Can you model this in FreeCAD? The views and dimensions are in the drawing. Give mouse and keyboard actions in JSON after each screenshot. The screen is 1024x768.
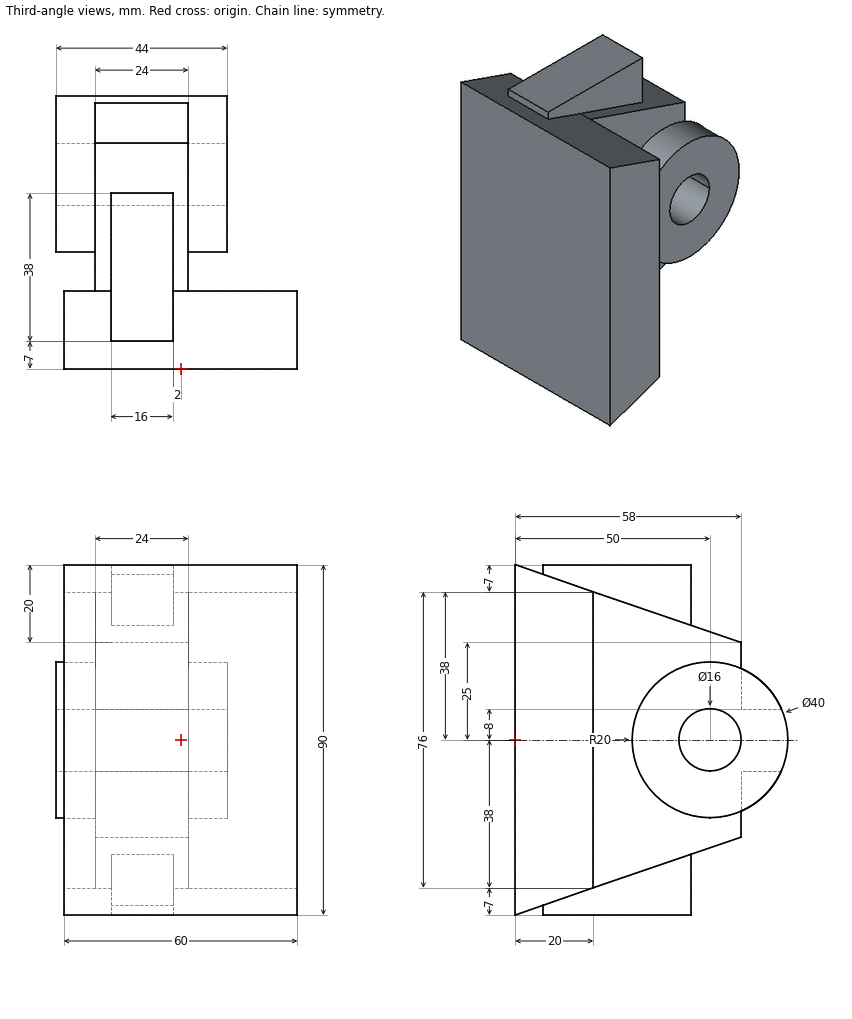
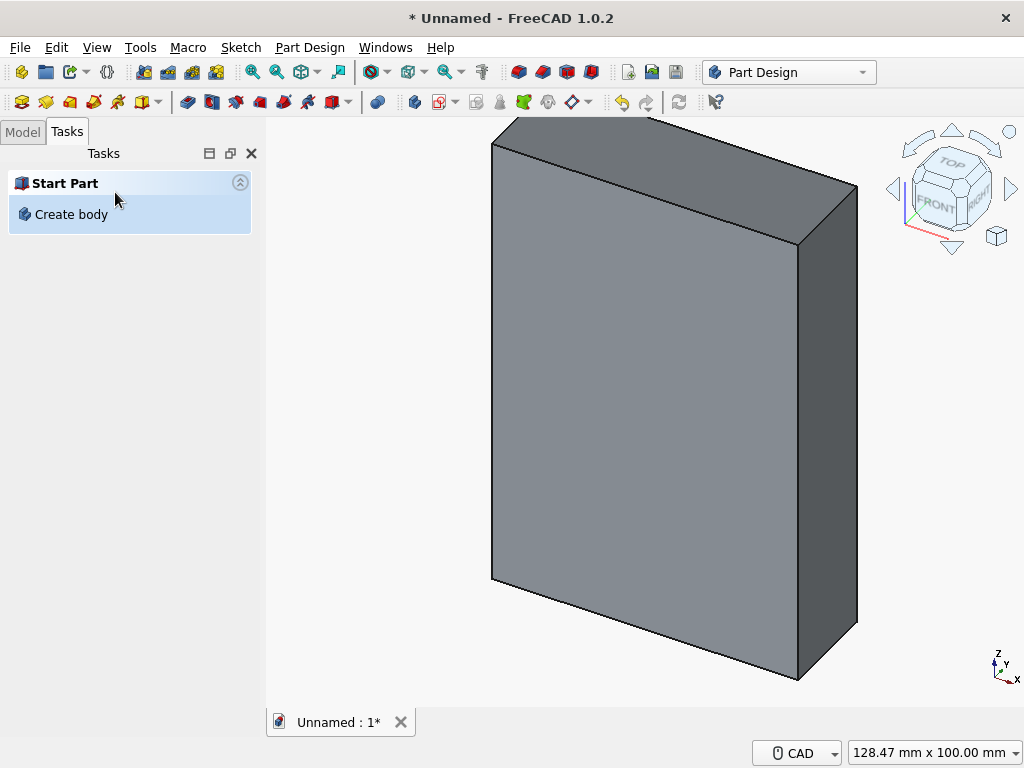
{"action": "left_click", "coordinate": [254, 72]}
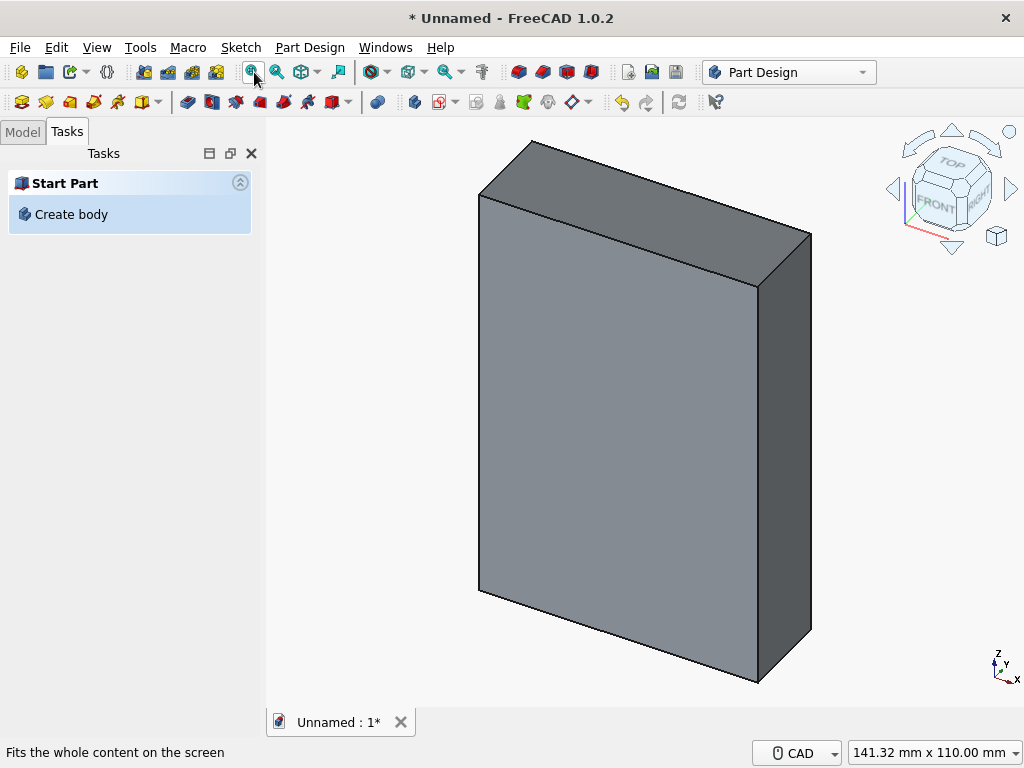
{"action": "left_click", "coordinate": [784, 457]}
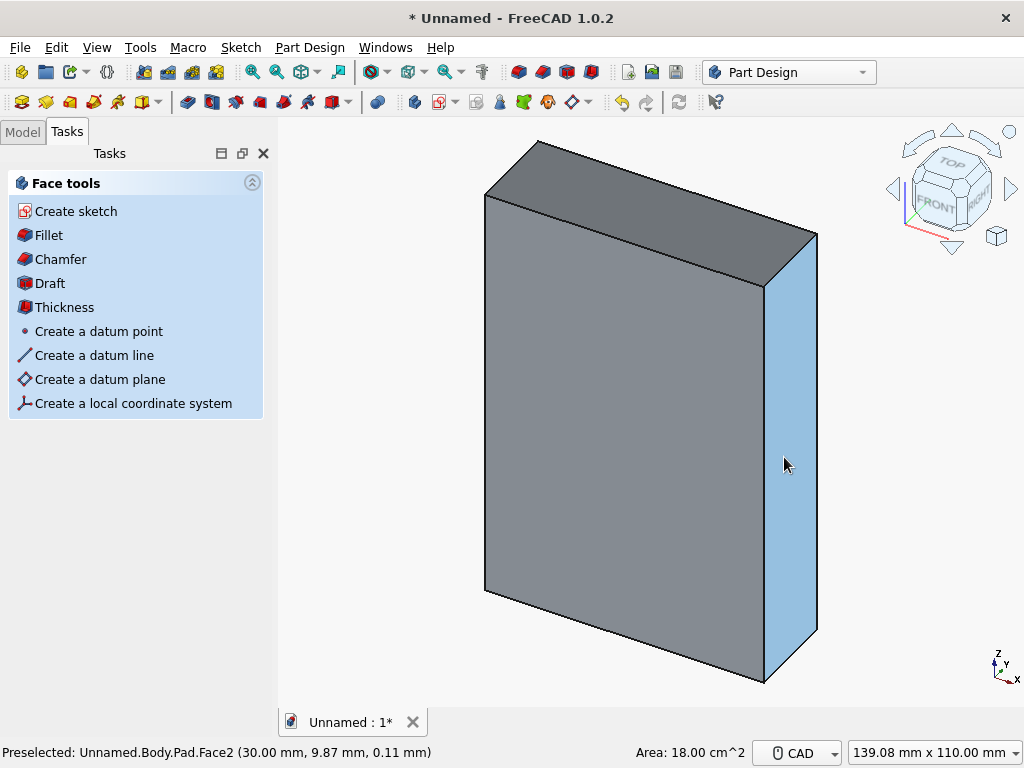
{"action": "left_click", "coordinate": [440, 102]}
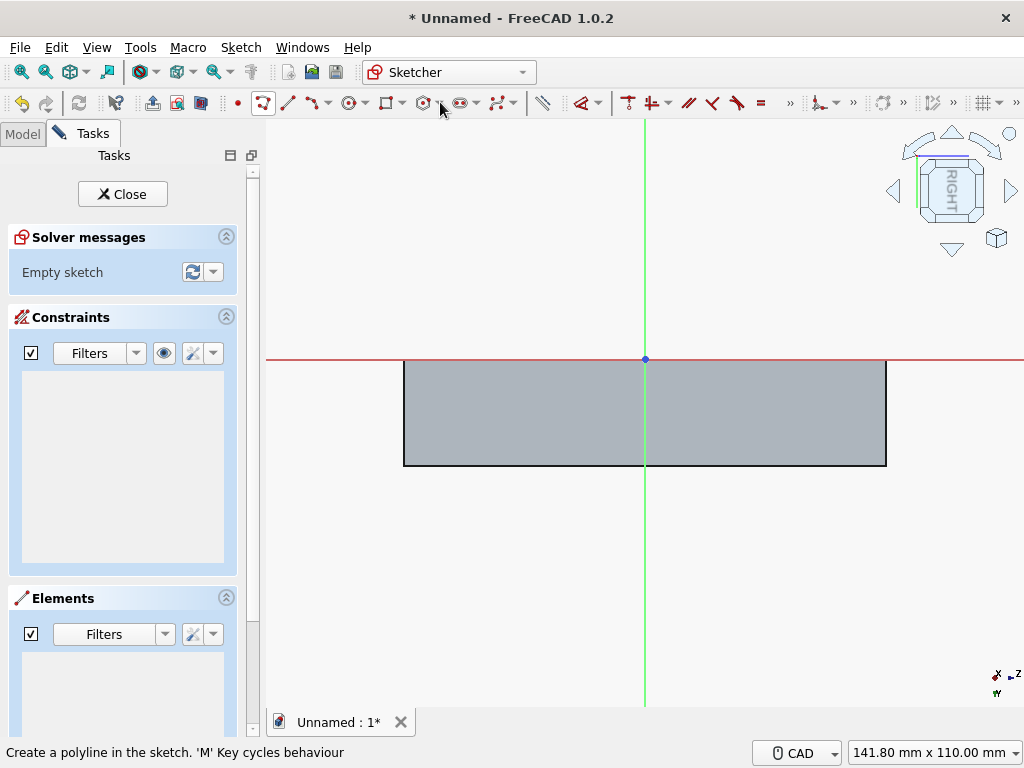
{"action": "scroll", "coordinate": [294, 413], "scroll_direction": "down", "scroll_amount": 1}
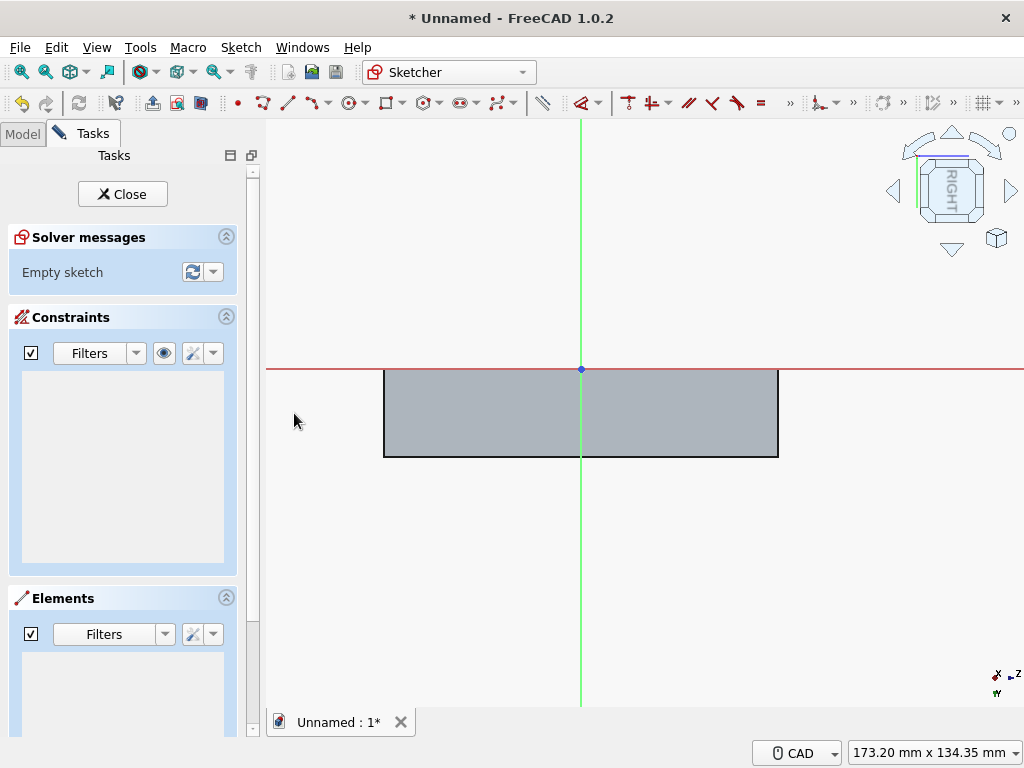
{"action": "left_click", "coordinate": [264, 104]}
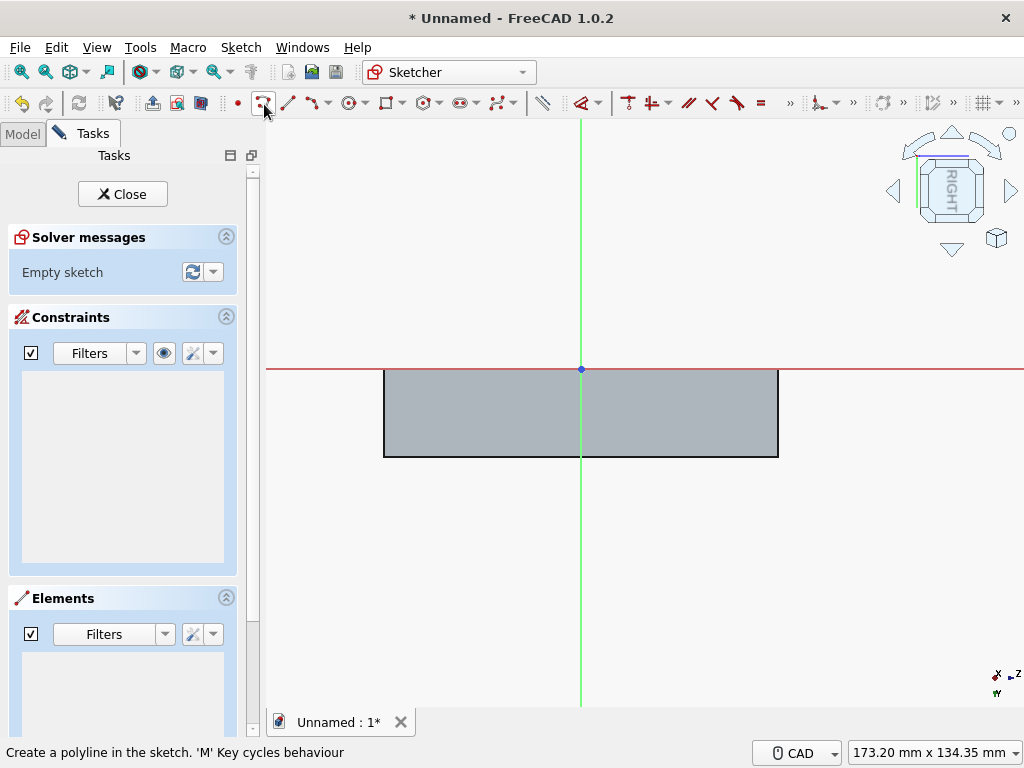
{"action": "left_click", "coordinate": [415, 457]}
{"action": "left_click", "coordinate": [384, 369]}
{"action": "left_click", "coordinate": [384, 457]}
{"action": "left_click", "coordinate": [415, 458]}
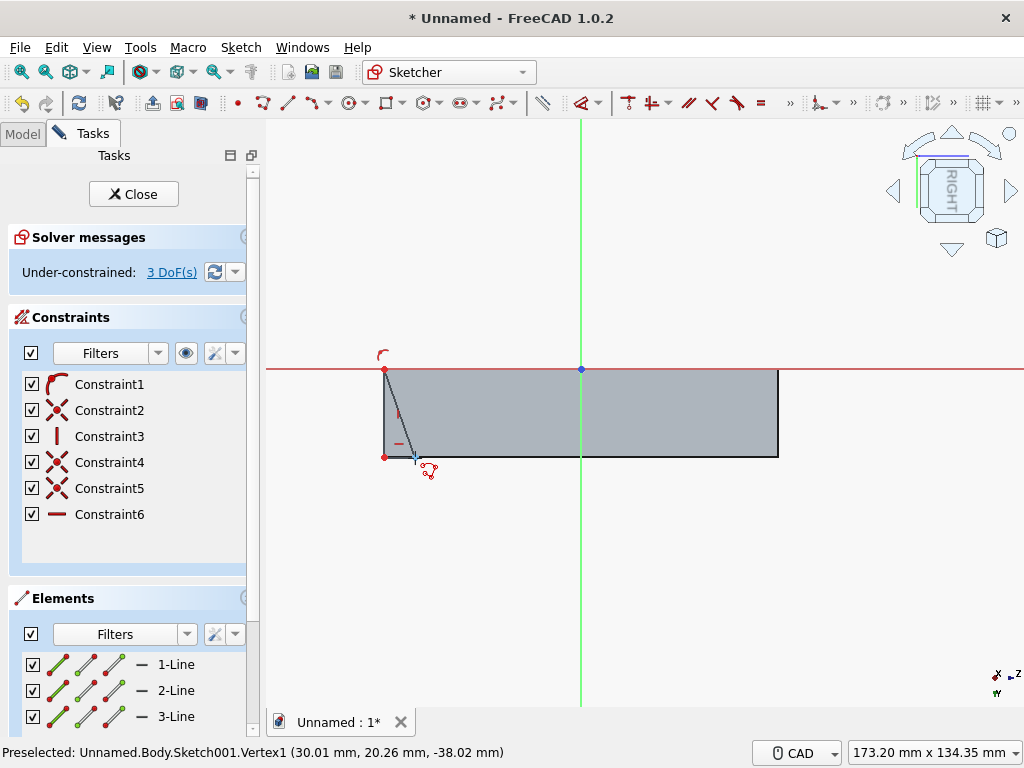
{"action": "left_click", "coordinate": [748, 457]}
{"action": "left_click", "coordinate": [778, 457]}
{"action": "left_click", "coordinate": [778, 369]}
{"action": "left_click", "coordinate": [748, 458]}
{"action": "key", "text": "Escape"}
{"action": "key", "text": "Escape"}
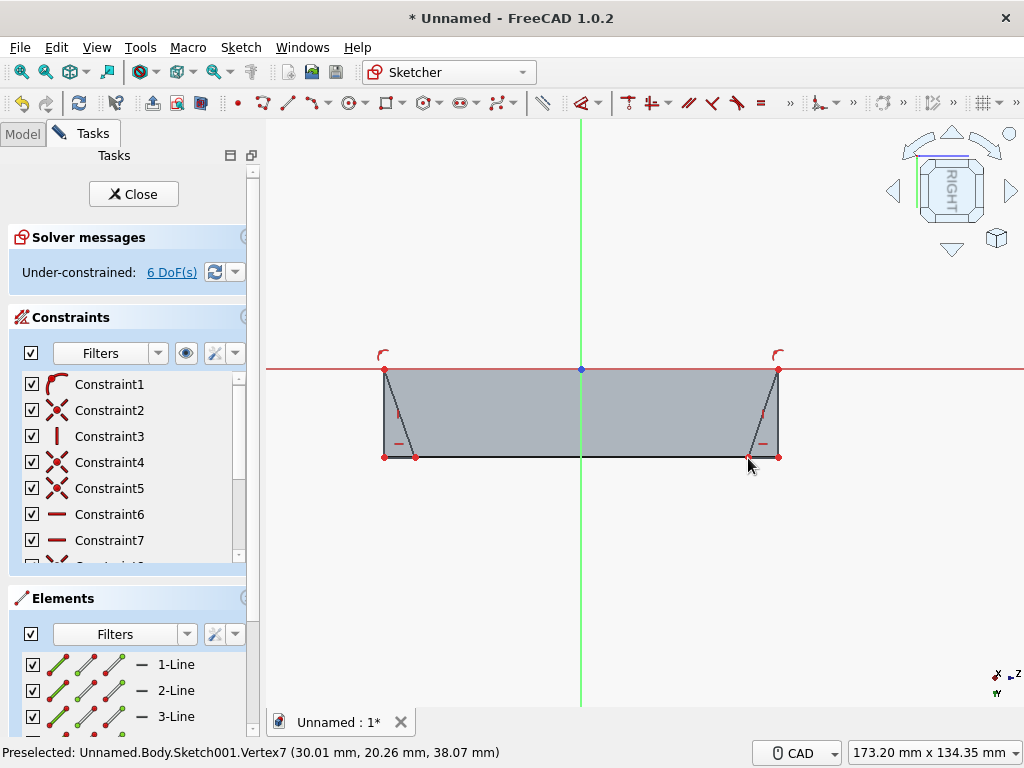
{"action": "left_click", "coordinate": [415, 458]}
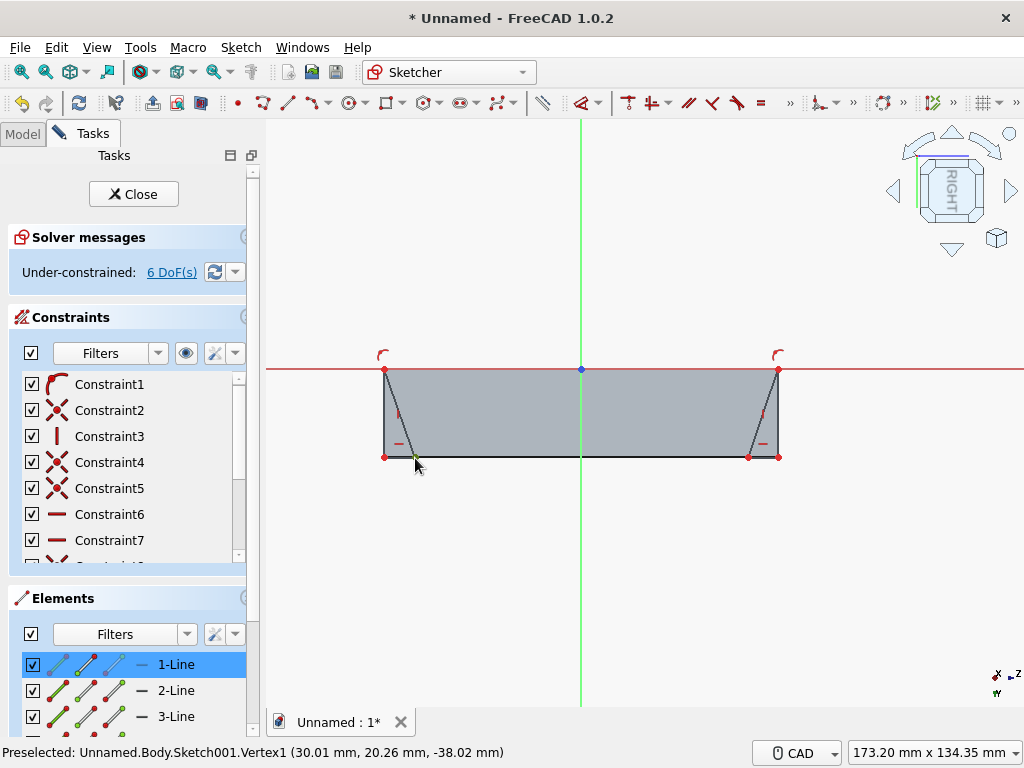
{"action": "left_click", "coordinate": [748, 458]}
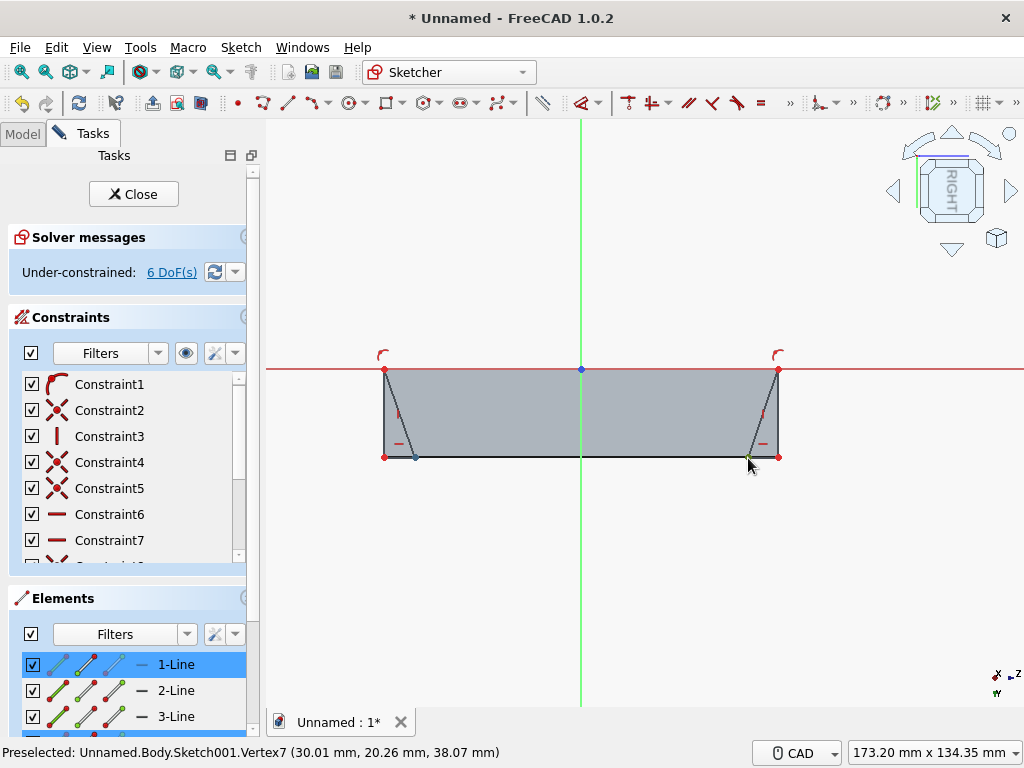
{"action": "left_click", "coordinate": [581, 641]}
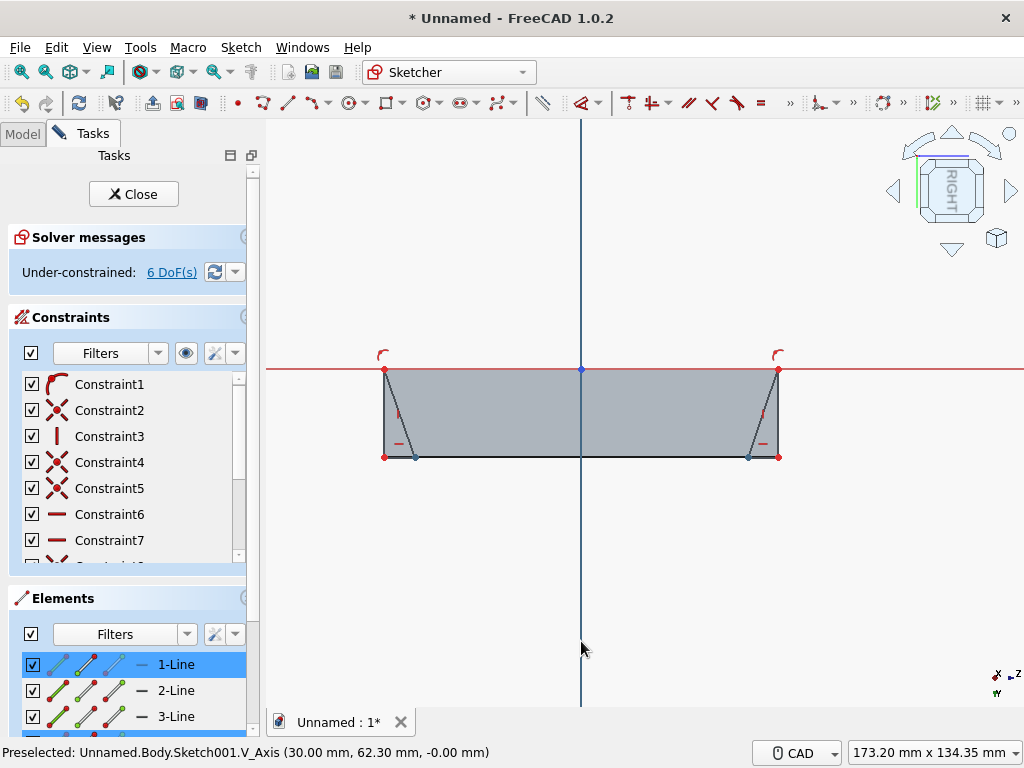
{"action": "key", "text": "s"}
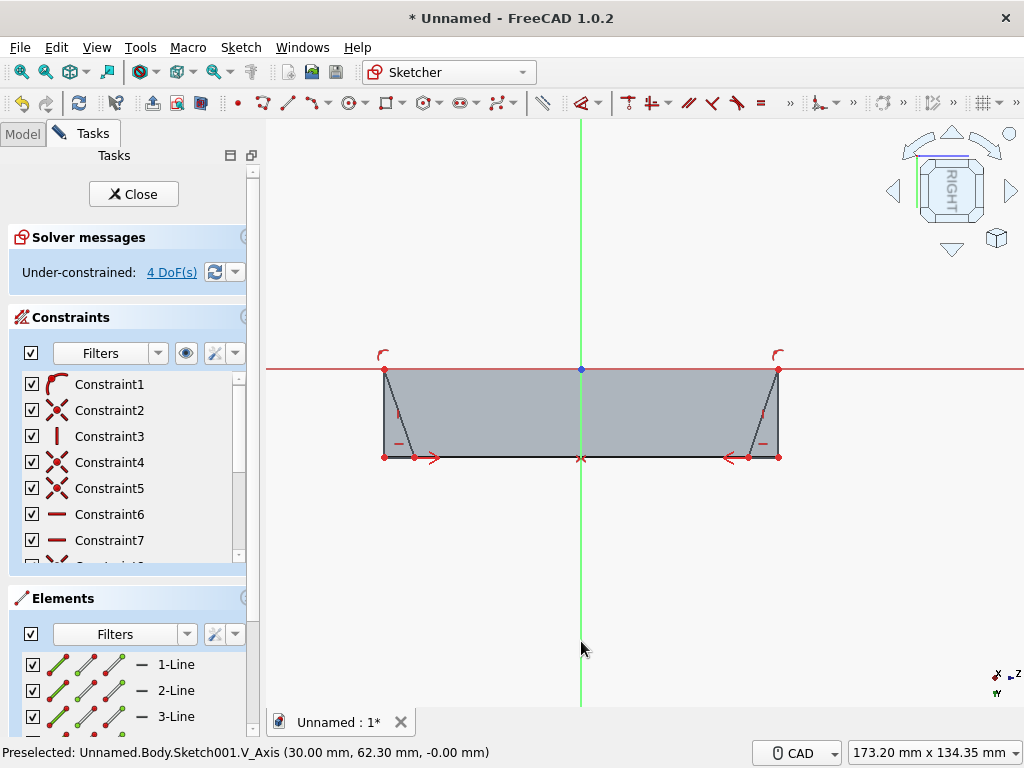
{"action": "left_click", "coordinate": [582, 104]}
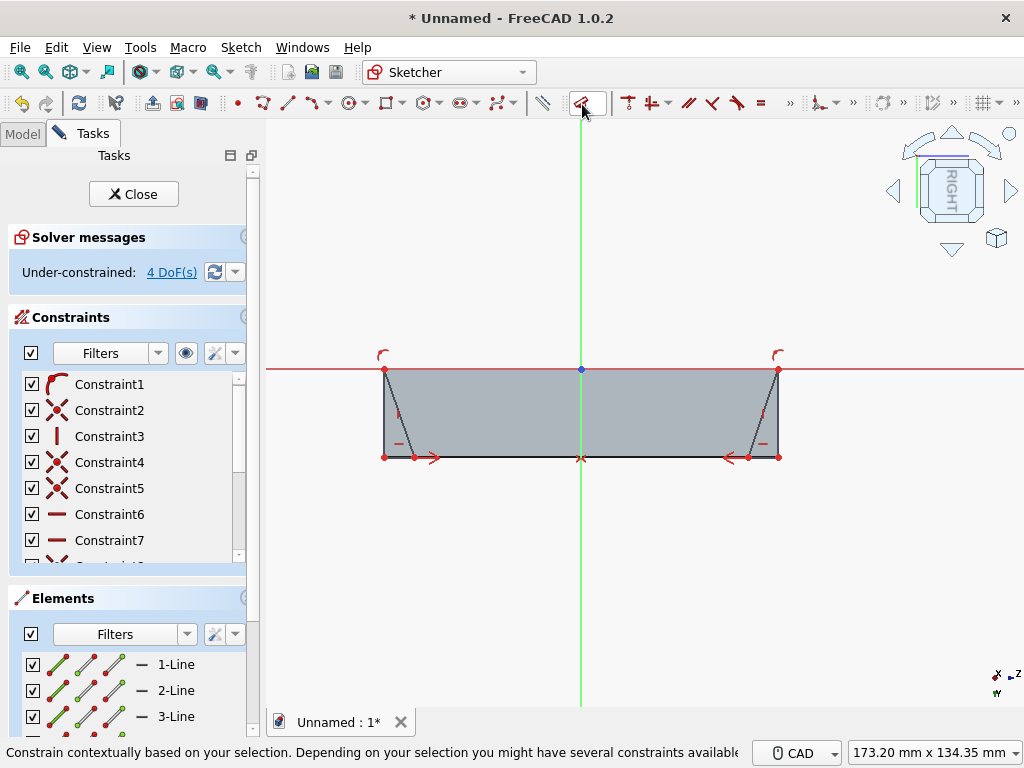
{"action": "scroll", "coordinate": [393, 458], "scroll_direction": "up", "scroll_amount": 3}